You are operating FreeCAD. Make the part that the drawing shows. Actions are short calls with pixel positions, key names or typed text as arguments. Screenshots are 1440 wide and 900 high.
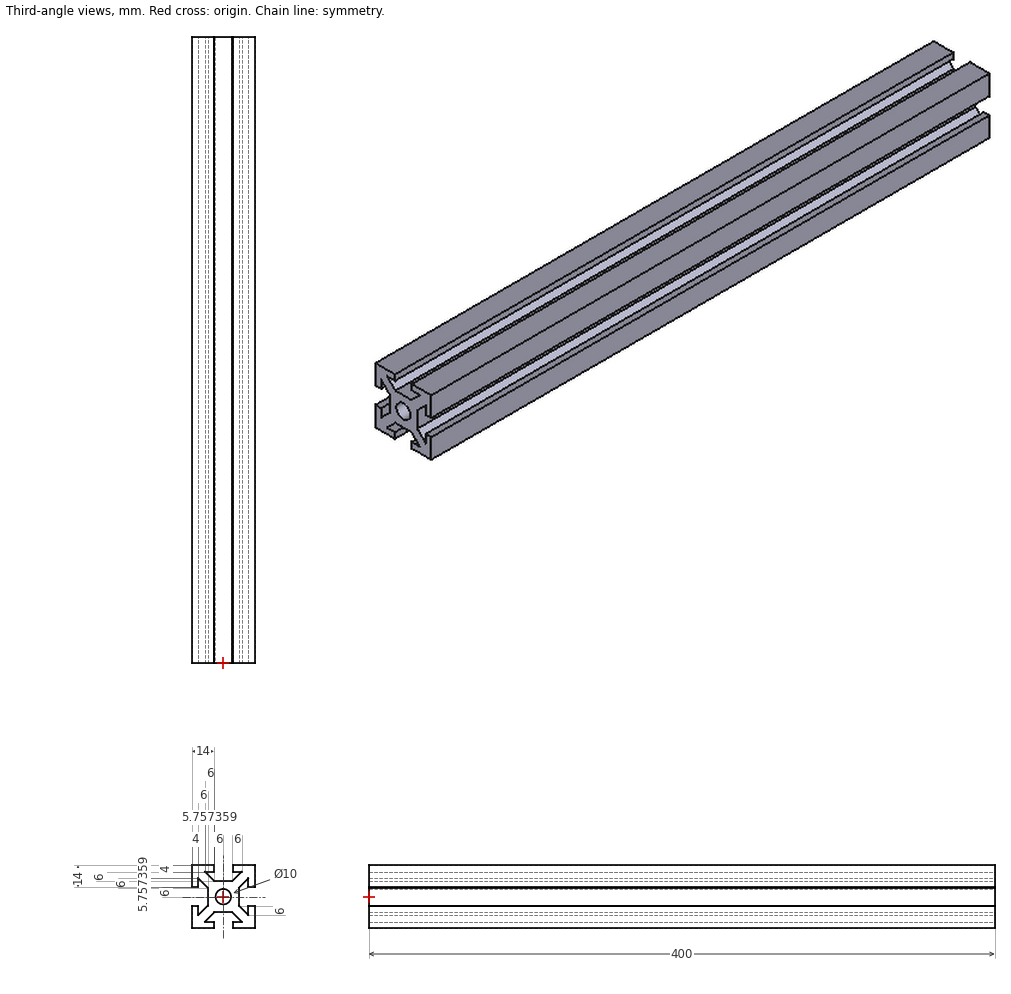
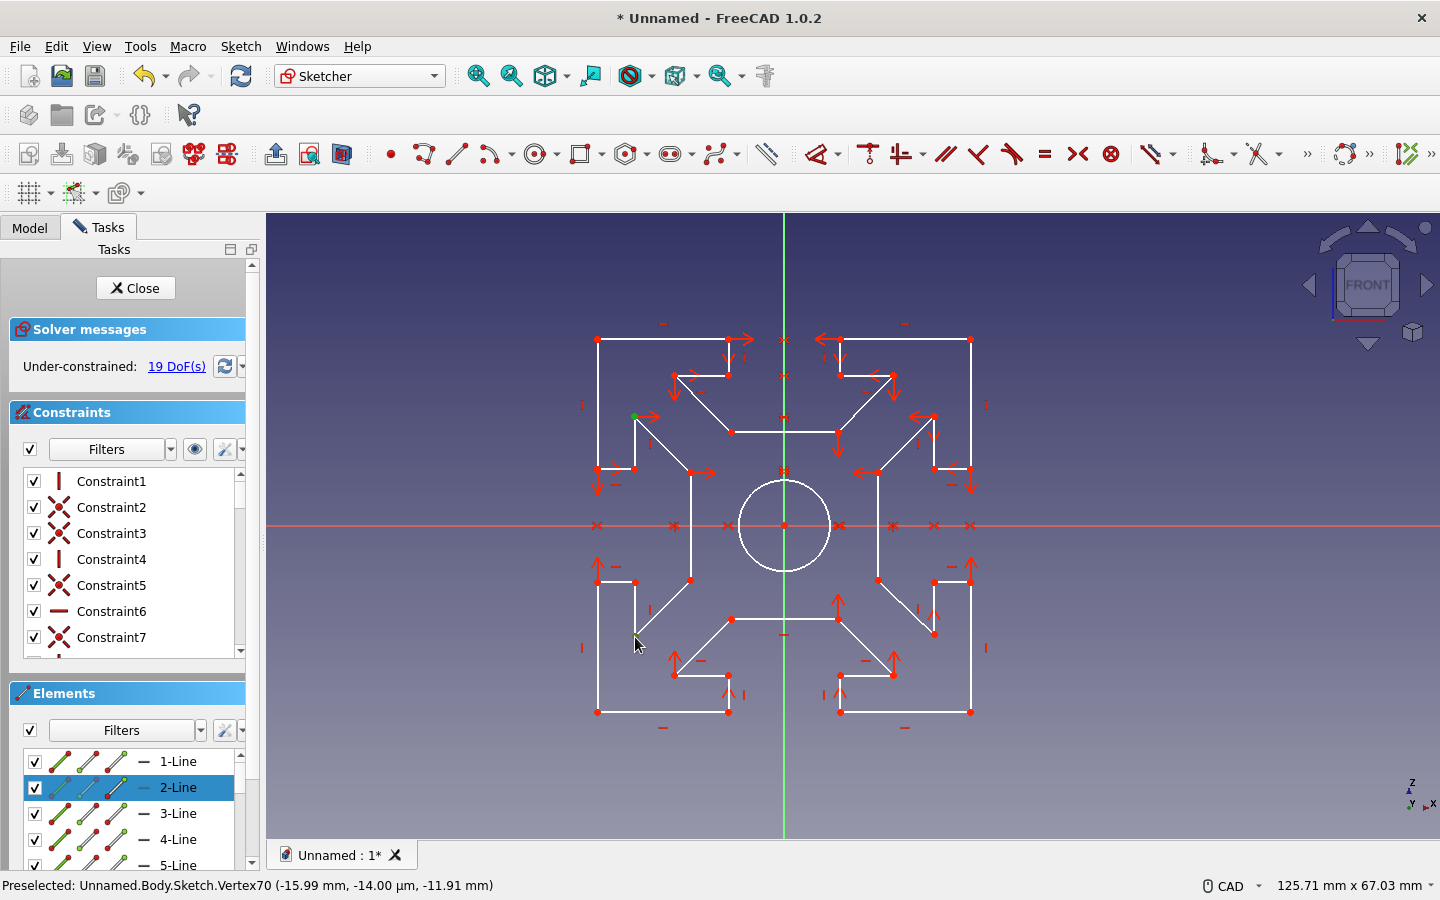
click(364, 526)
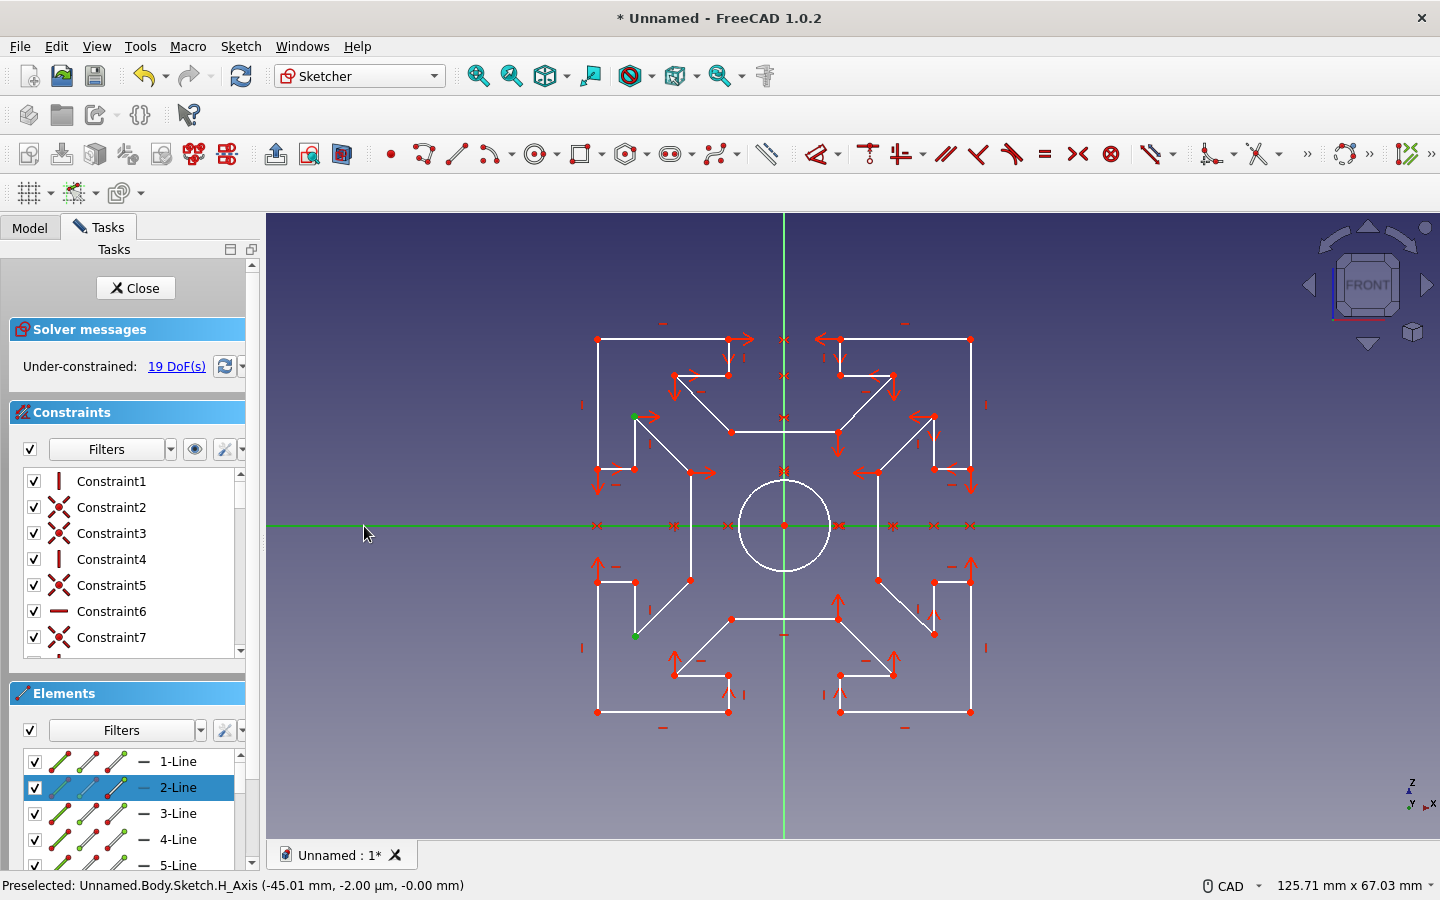
click(1078, 154)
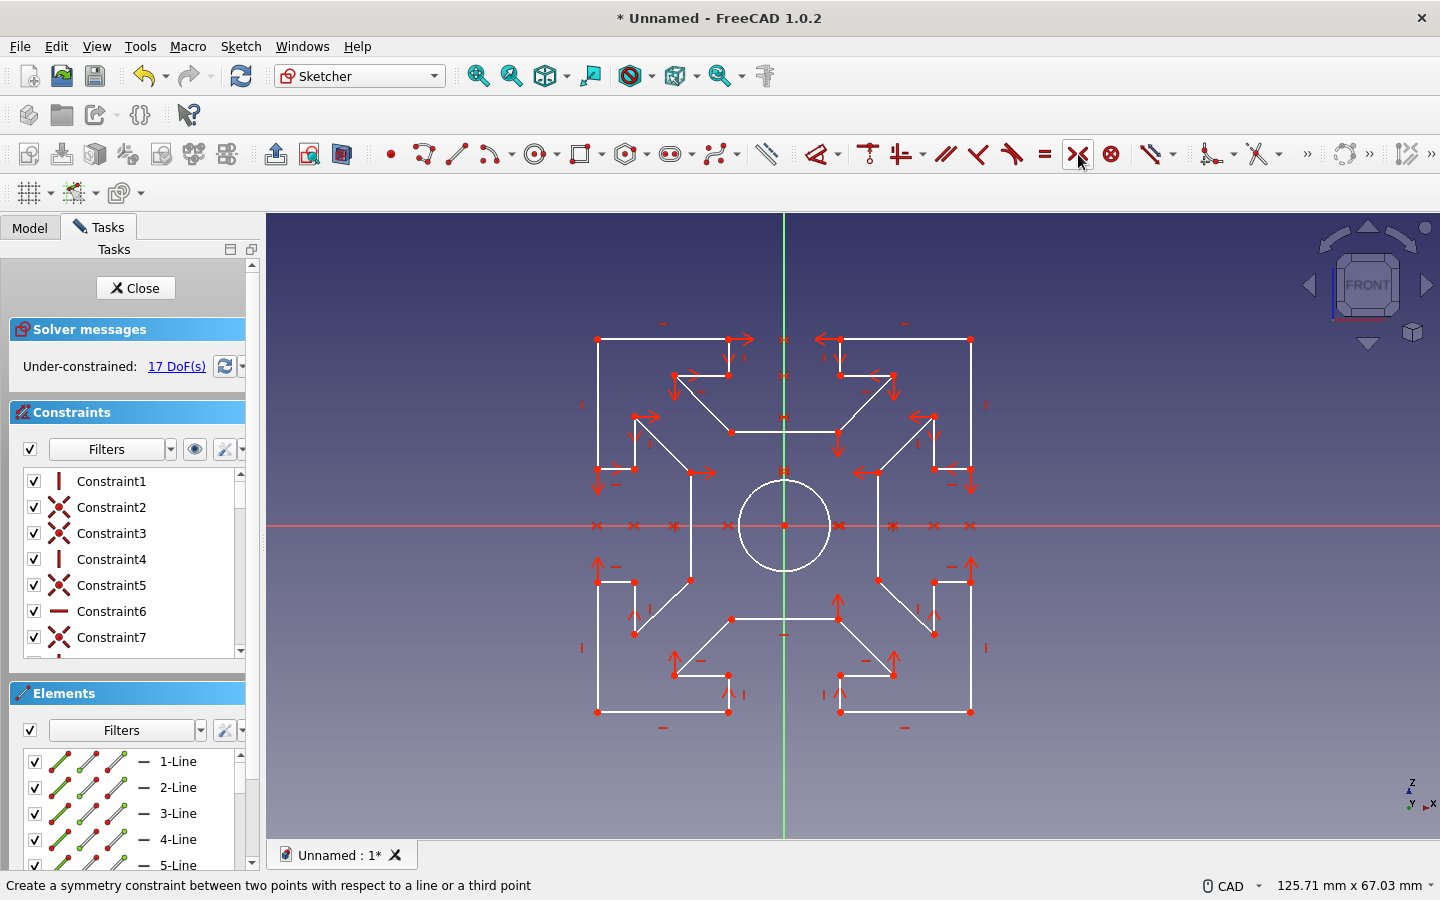
click(816, 493)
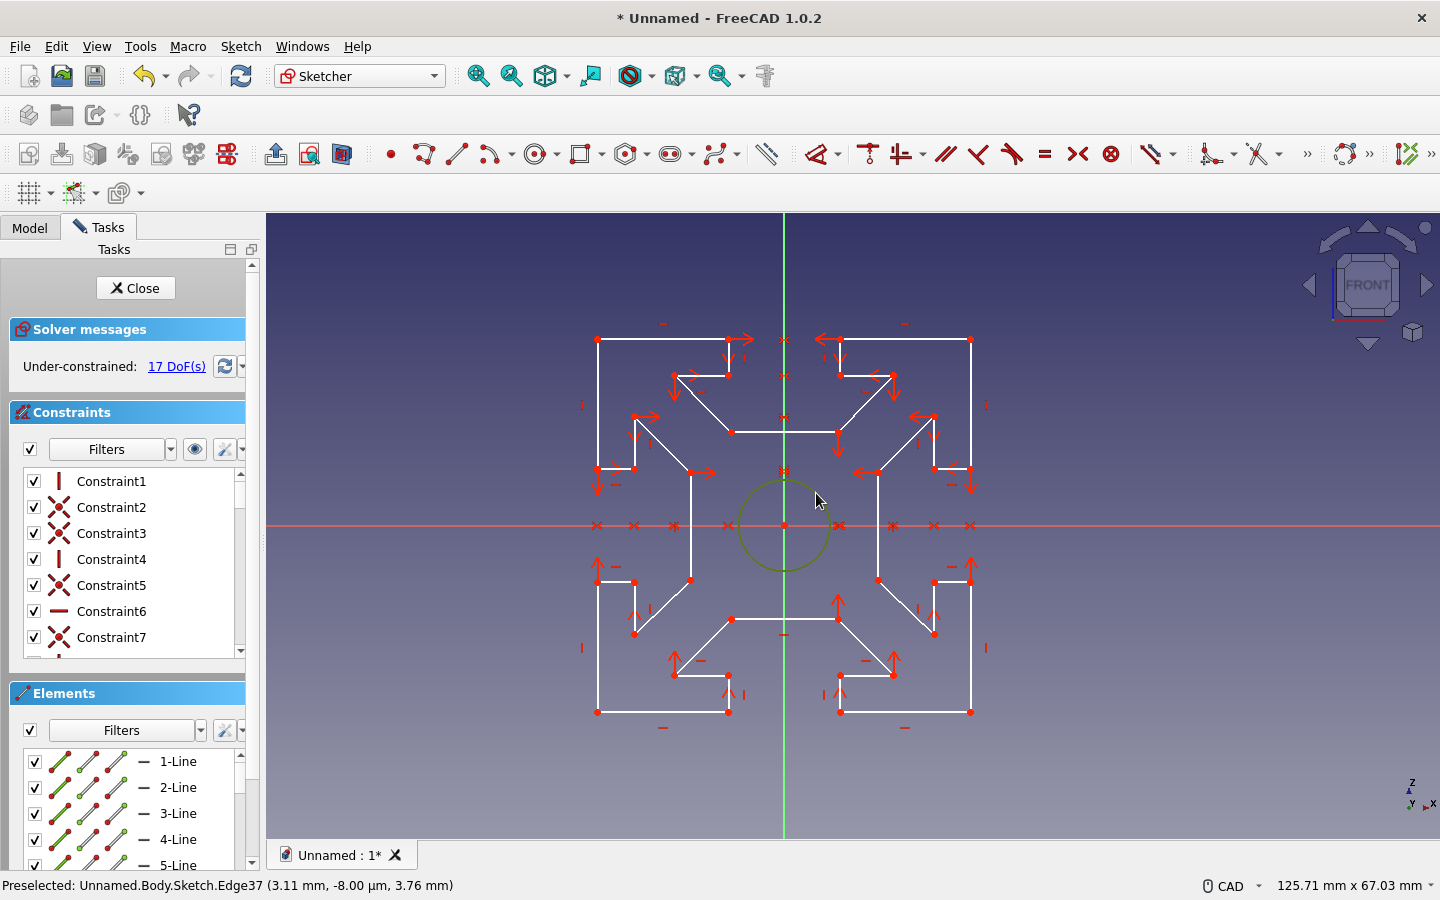
key(k)
key(o)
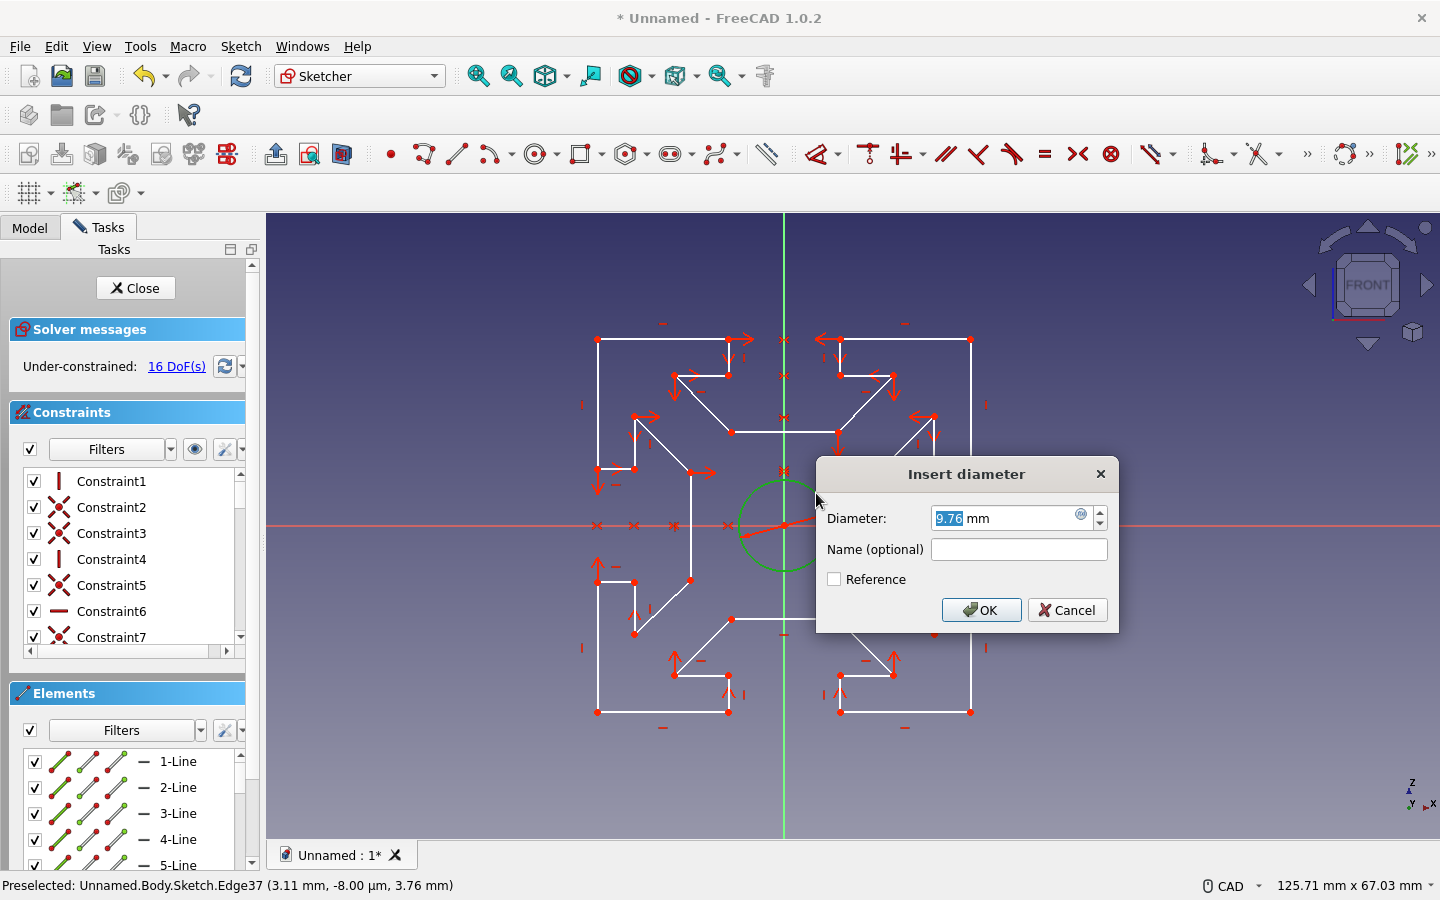
text(10)
key(Return)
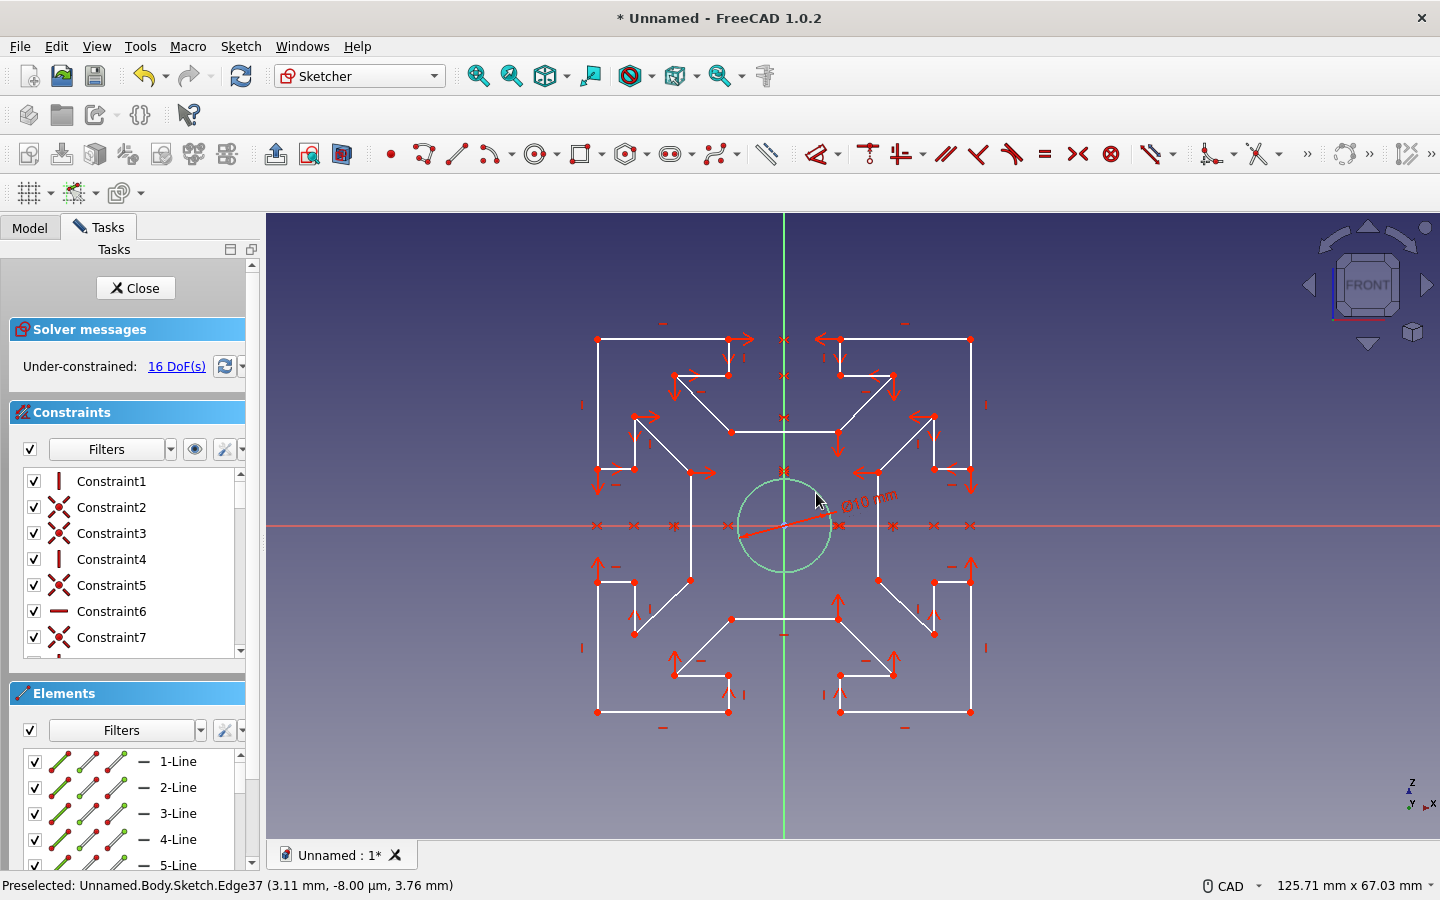
scroll(624, 469, up, 2)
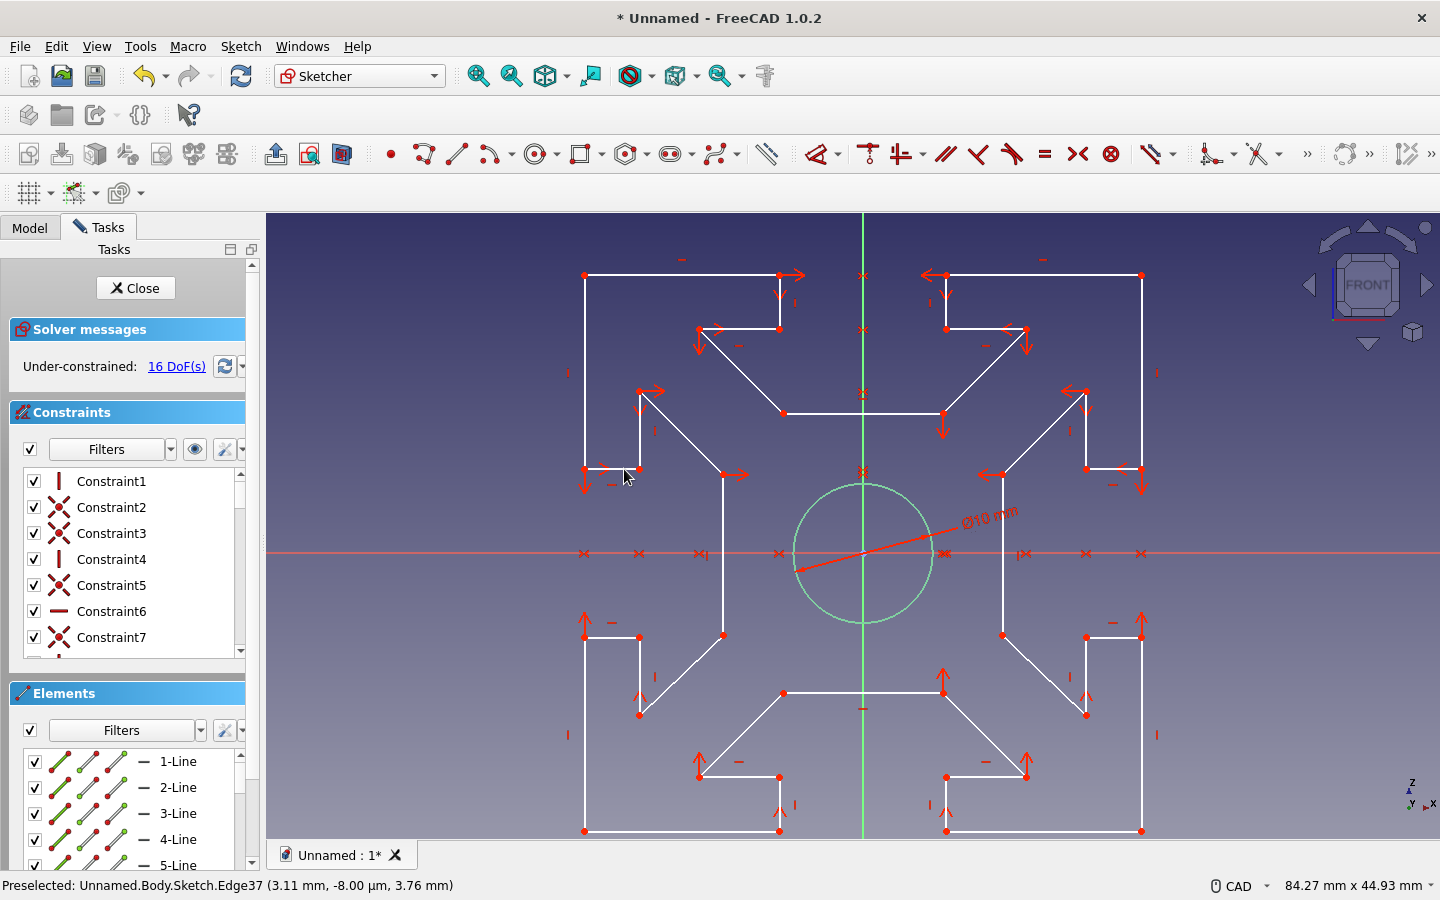
click(623, 469)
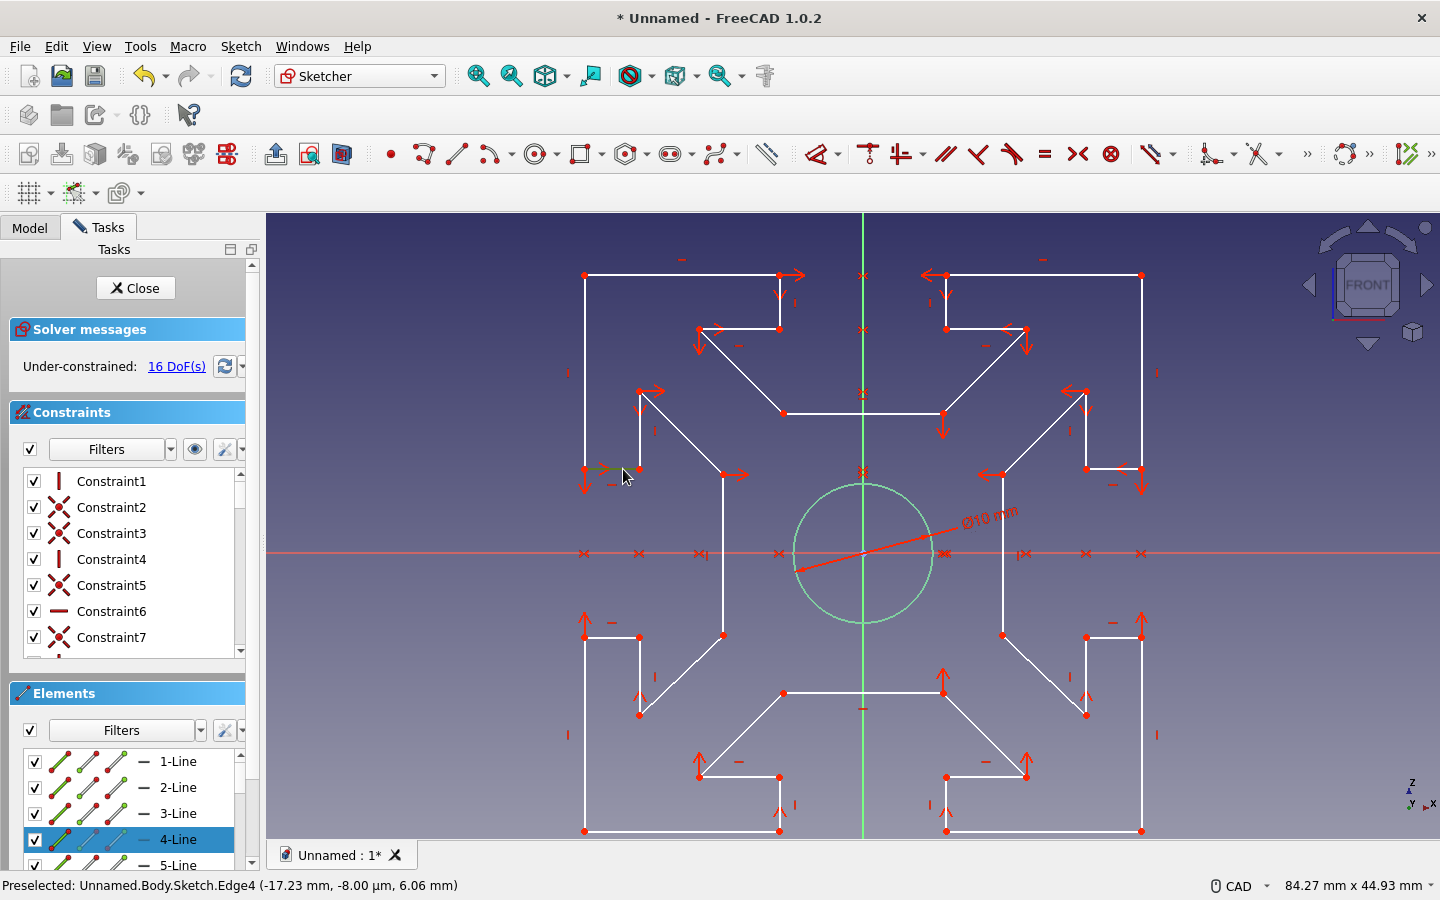
key(l)